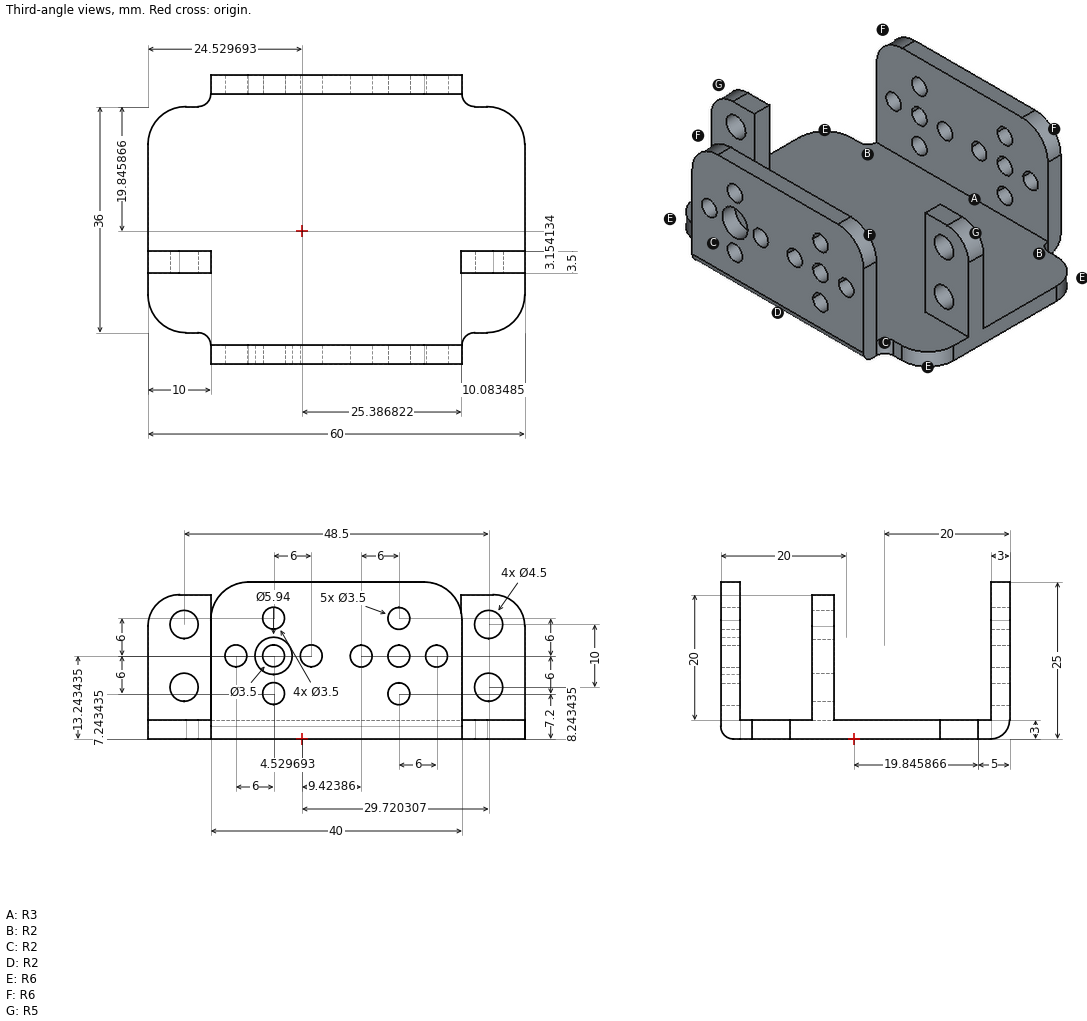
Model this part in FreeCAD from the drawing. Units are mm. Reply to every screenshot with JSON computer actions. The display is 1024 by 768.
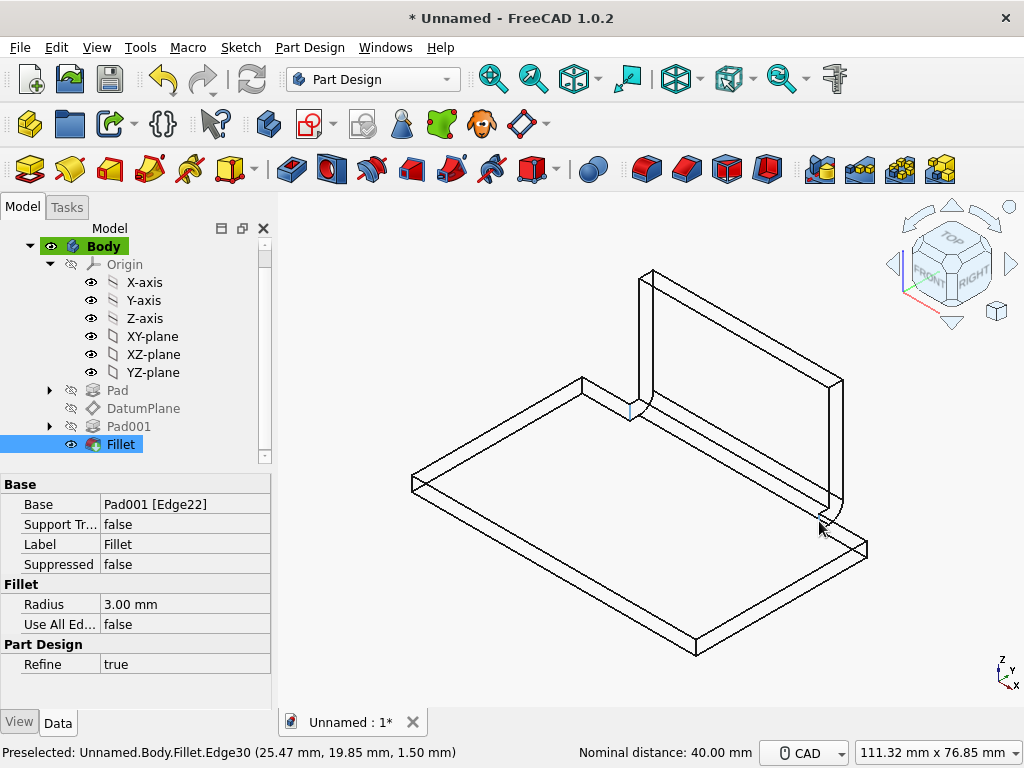
{"action": "key", "text": "v 1"}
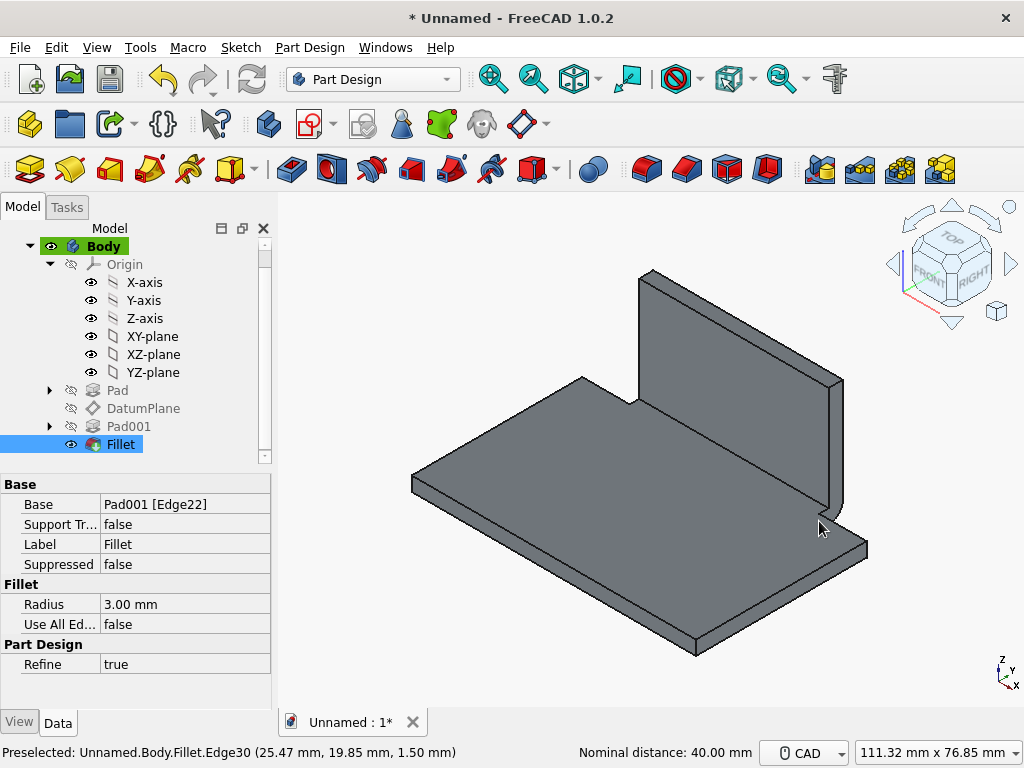
{"action": "left_click", "coordinate": [648, 170]}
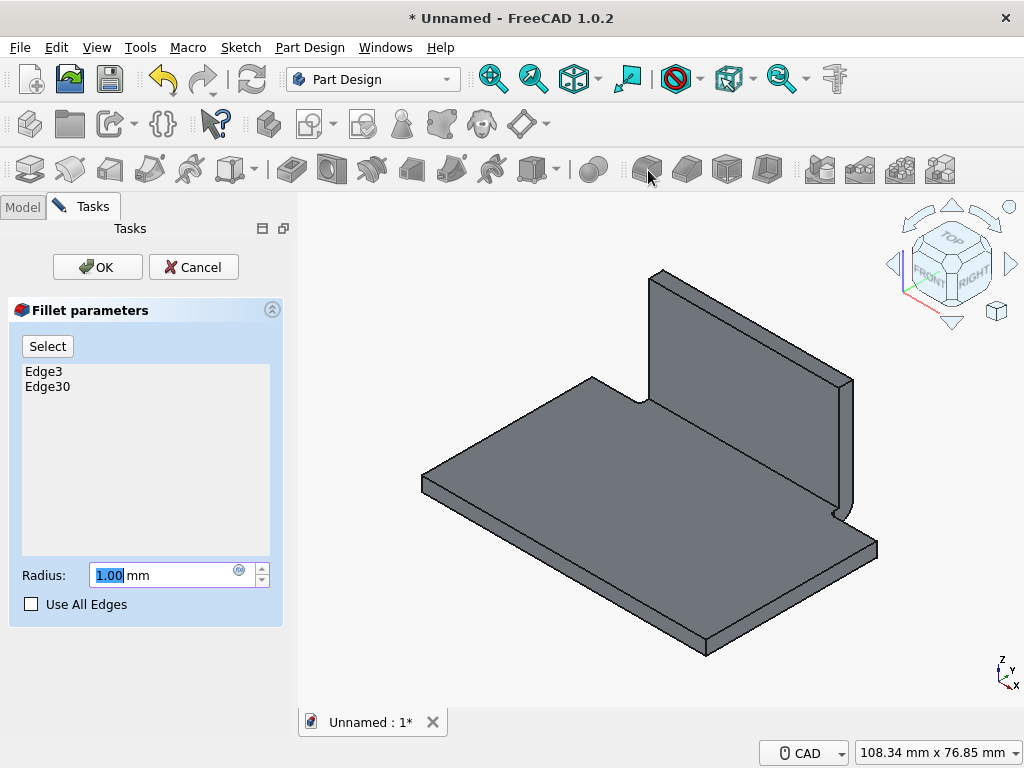
{"action": "type", "text": "2"}
{"action": "key", "text": "Tab"}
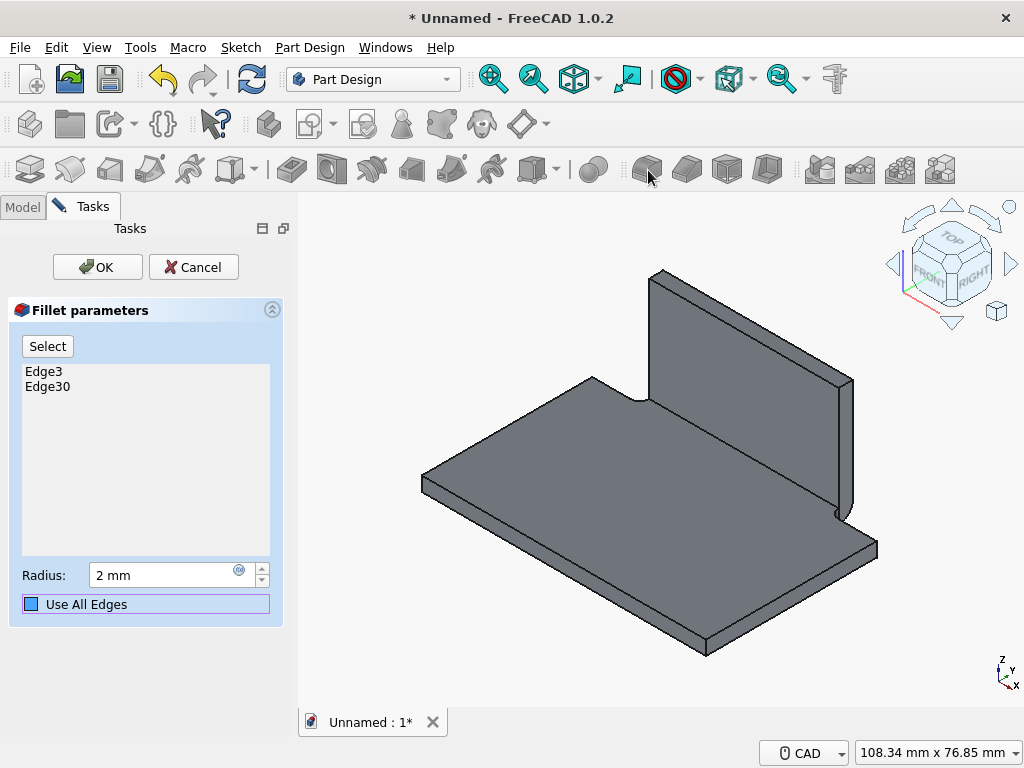
{"action": "left_click", "coordinate": [98, 267]}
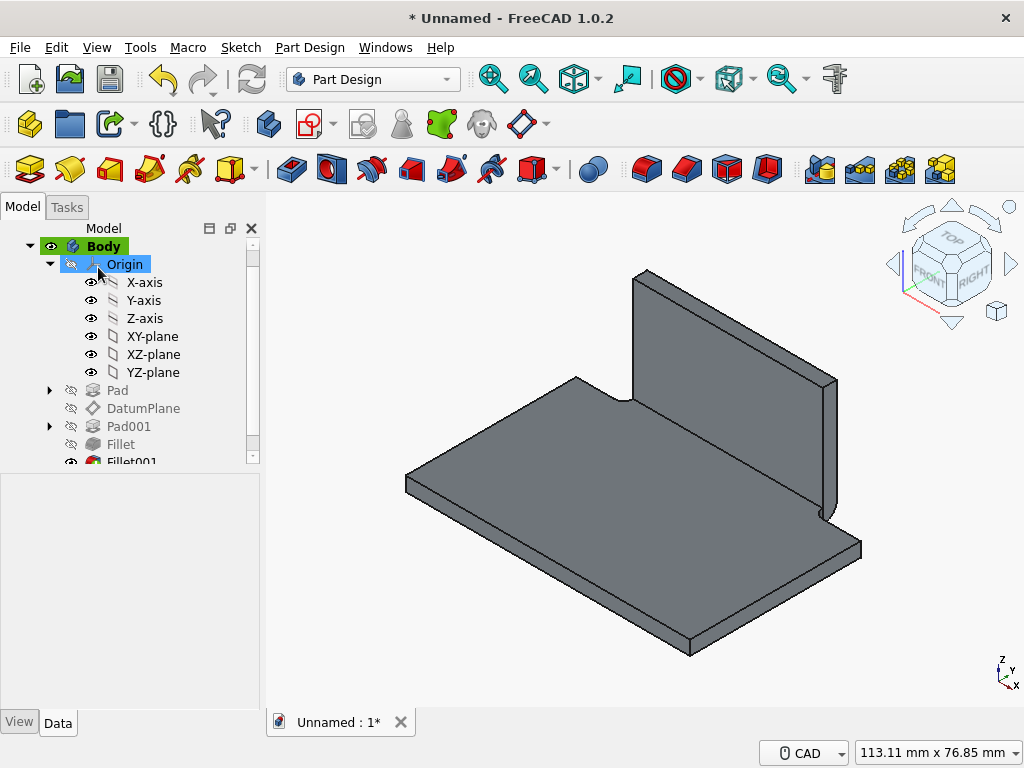
{"action": "left_click", "coordinate": [136, 354]}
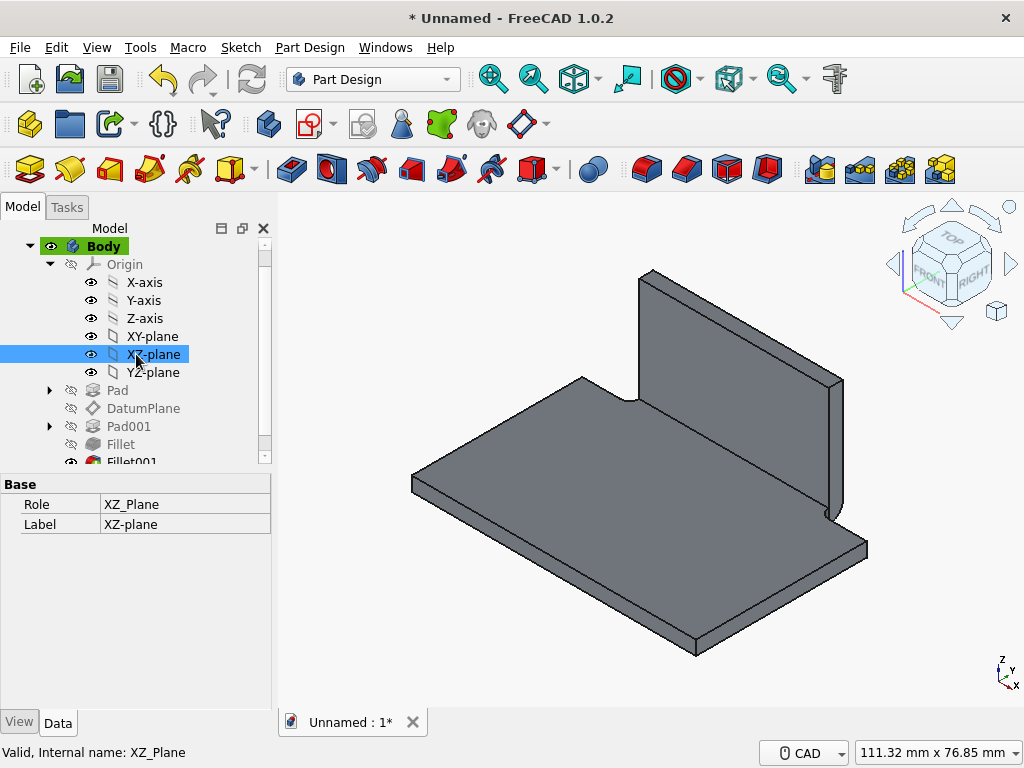
{"action": "left_click", "coordinate": [522, 124]}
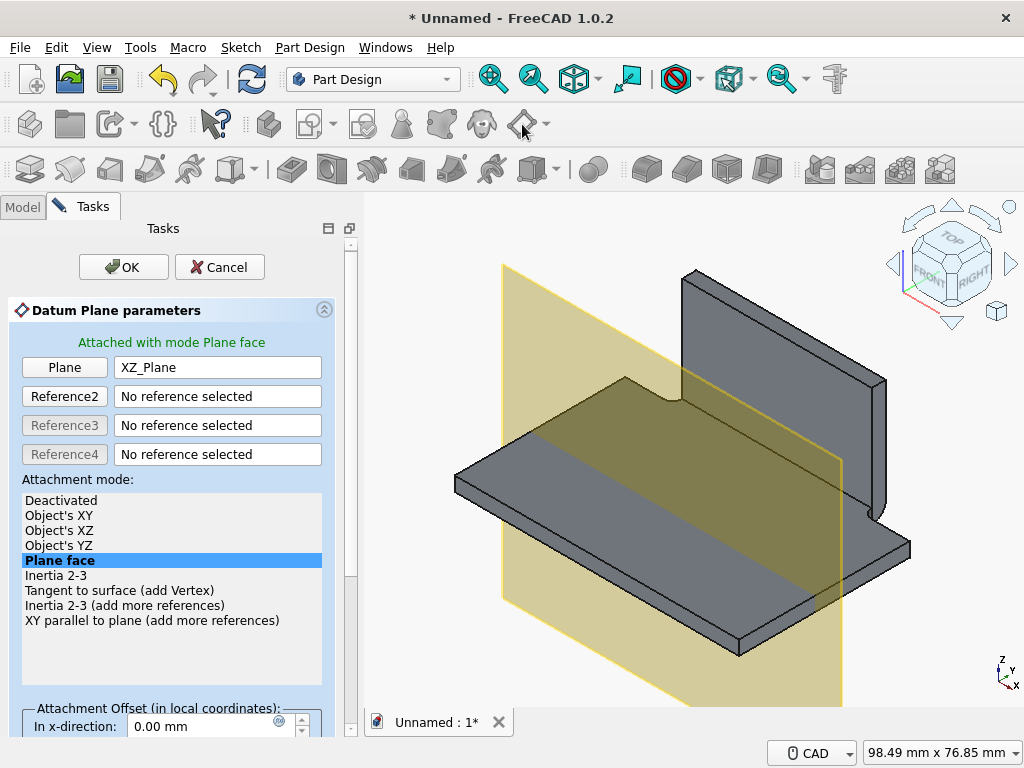
{"action": "scroll", "coordinate": [351, 487], "scroll_direction": "down", "scroll_amount": 3}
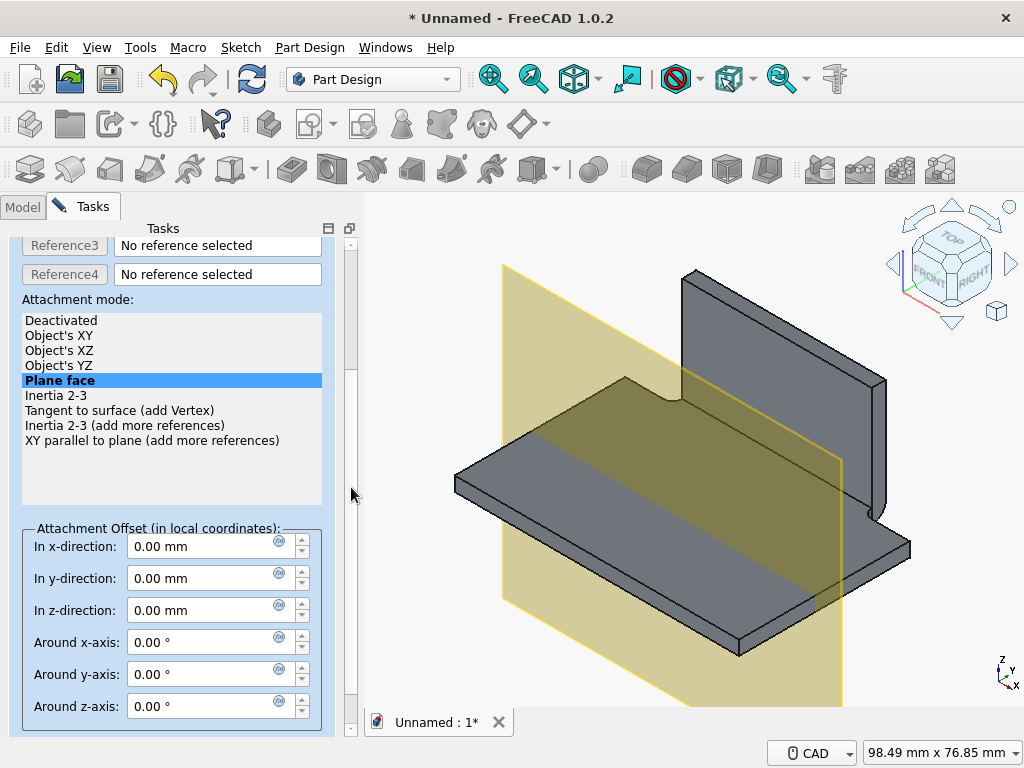
{"action": "triple_click", "coordinate": [210, 610]}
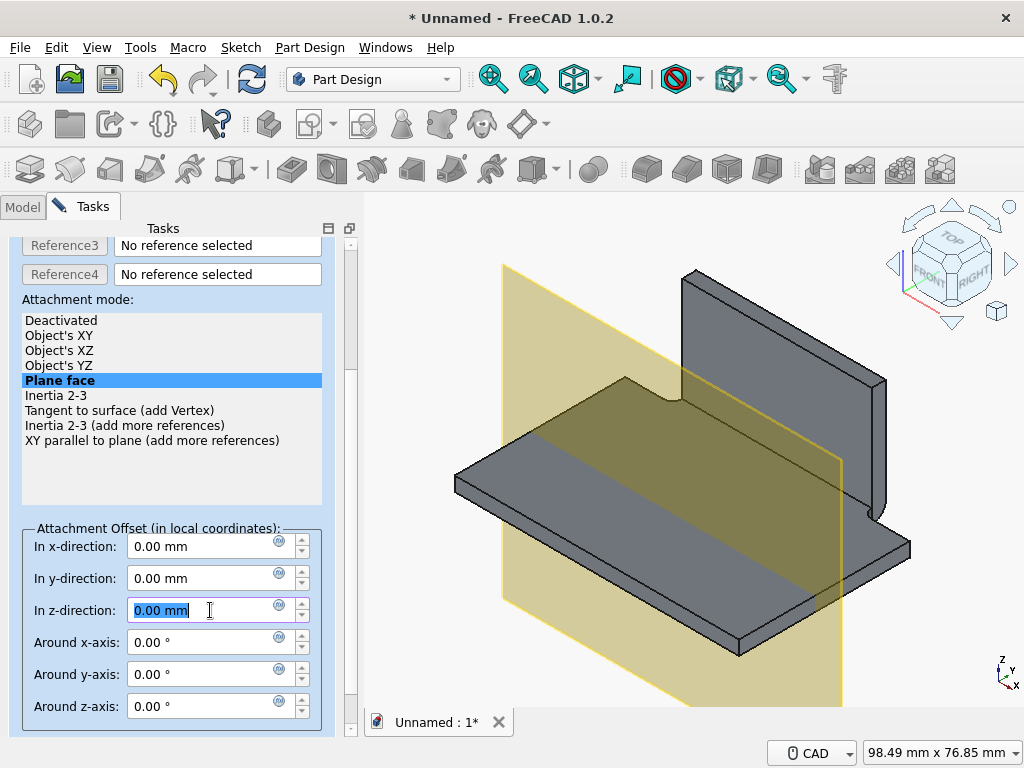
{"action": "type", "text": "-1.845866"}
{"action": "key", "text": "Tab"}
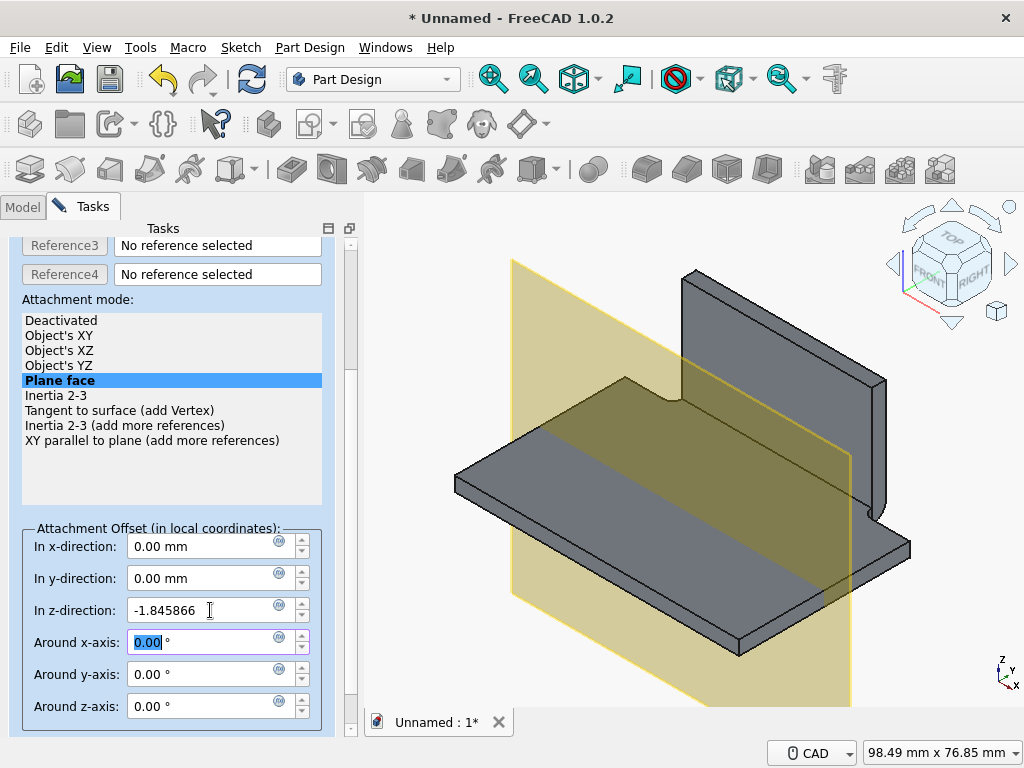
{"action": "scroll", "coordinate": [351, 487], "scroll_direction": "up", "scroll_amount": 4}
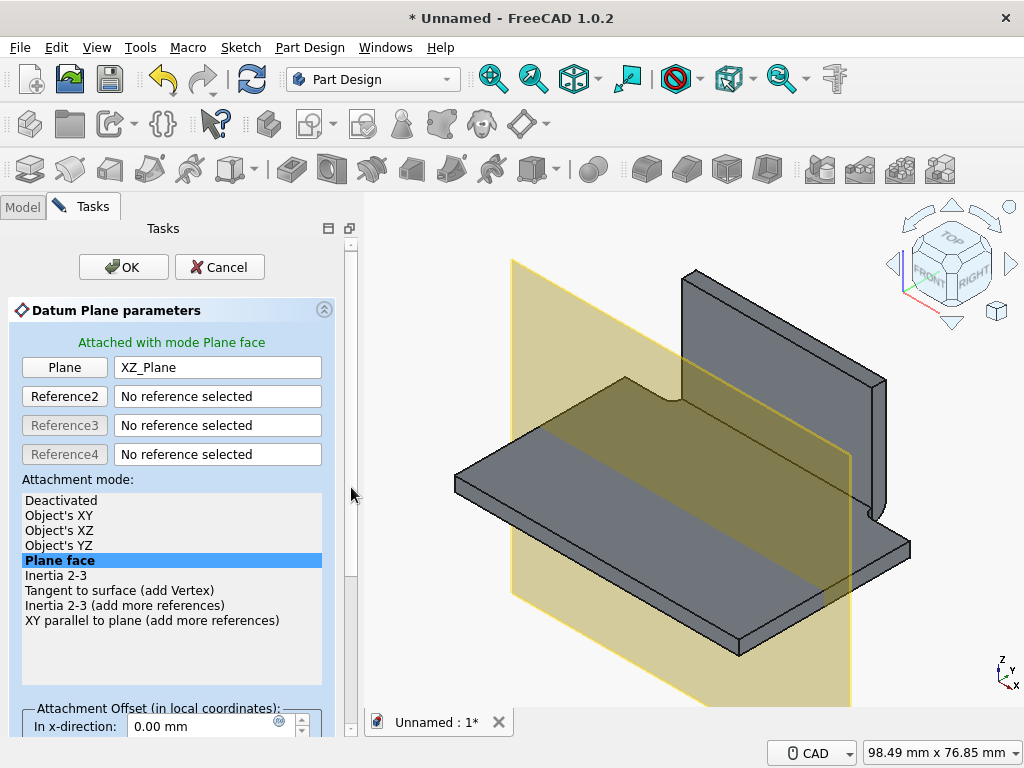
{"action": "left_click", "coordinate": [124, 267]}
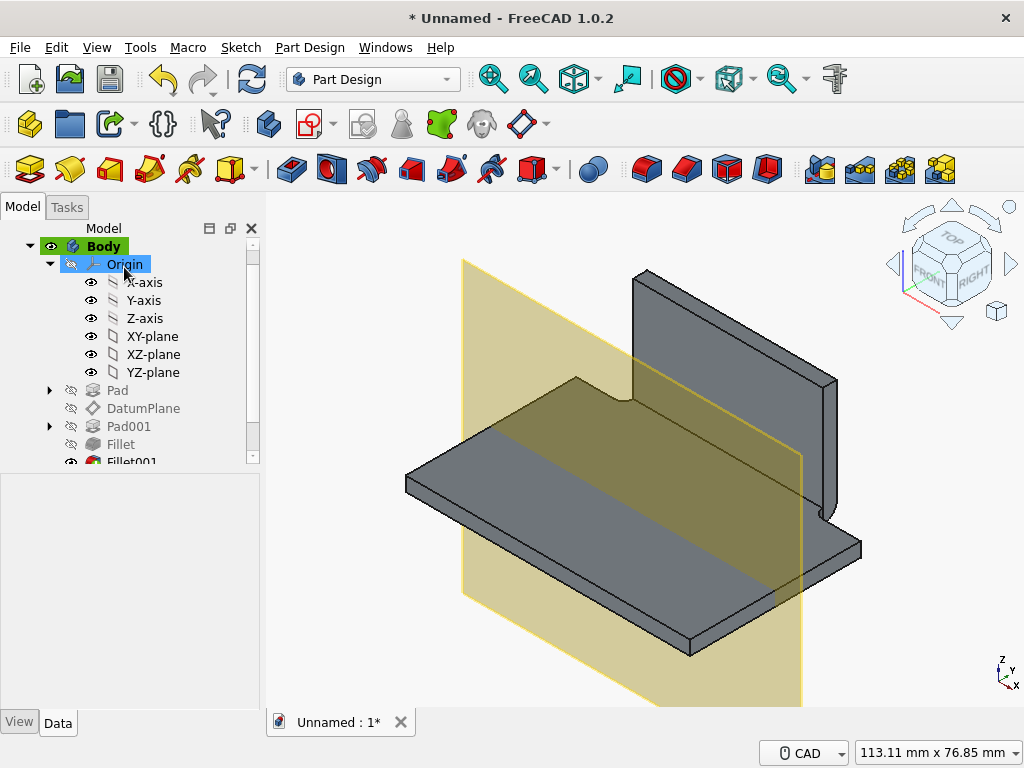
{"action": "left_click", "coordinate": [116, 426]}